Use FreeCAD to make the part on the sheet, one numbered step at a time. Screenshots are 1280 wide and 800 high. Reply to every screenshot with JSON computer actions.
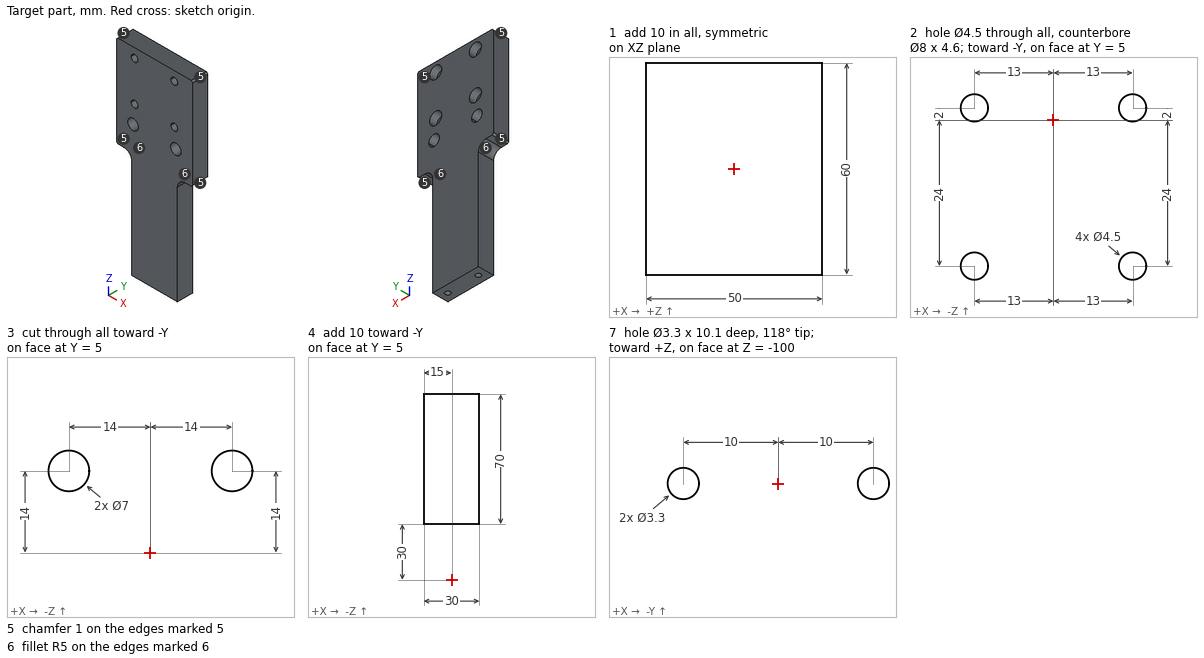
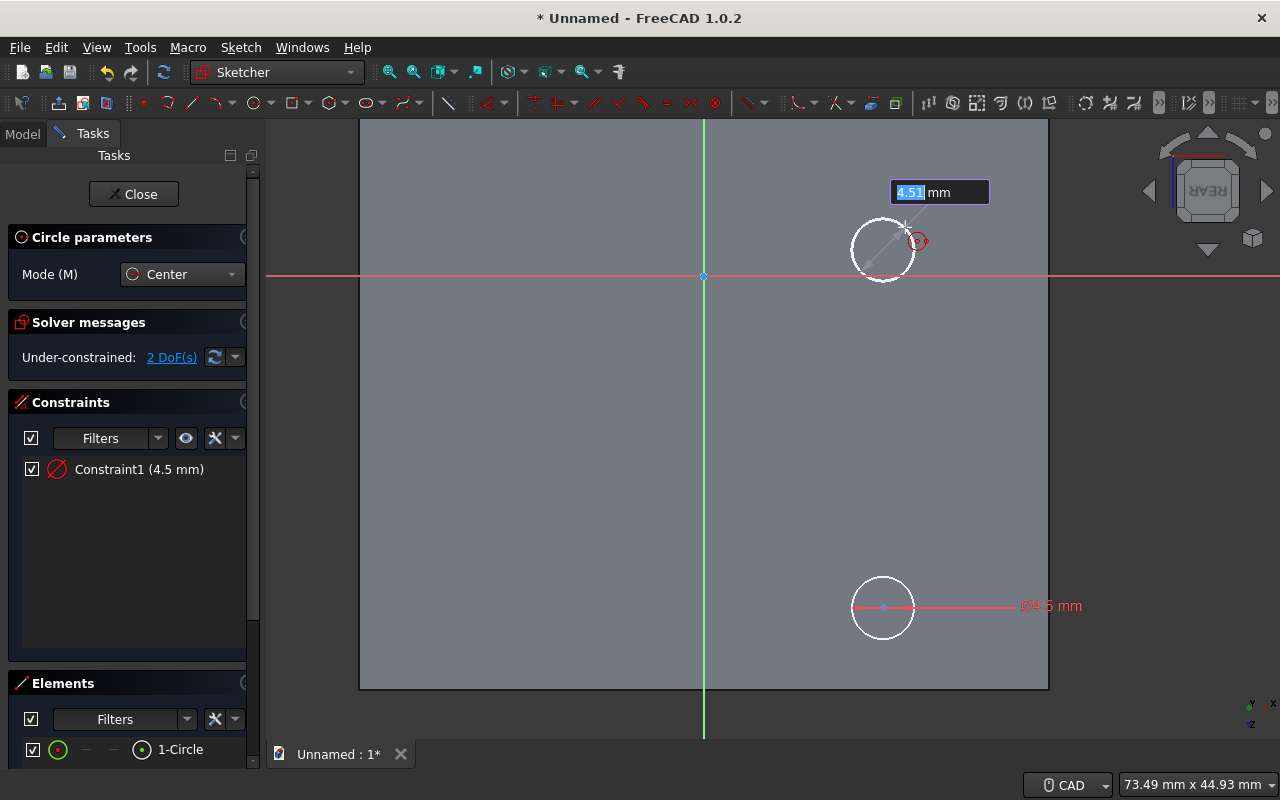
{"action": "type", "text": "4.5"}
{"action": "key", "text": "Return"}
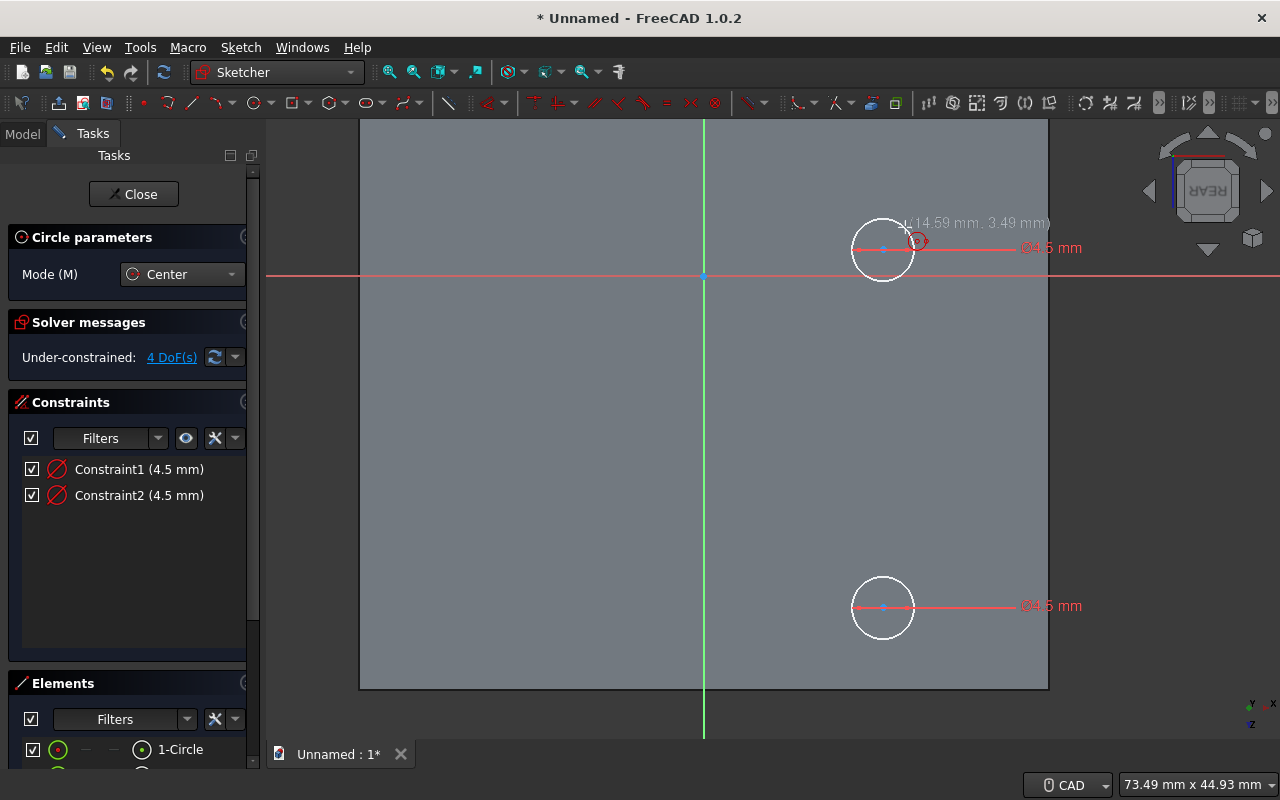
{"action": "left_click", "coordinate": [524, 249]}
{"action": "mouse_move", "coordinate": [546, 227]}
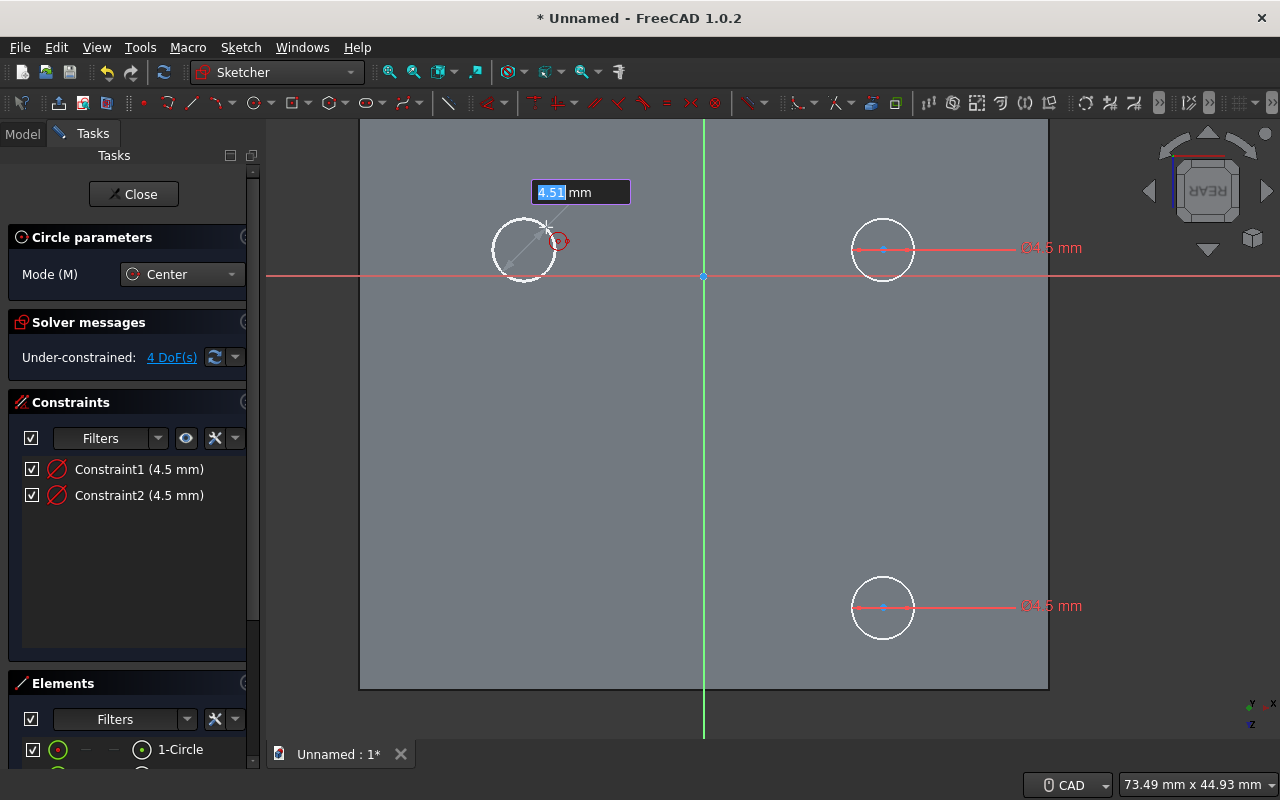
{"action": "type", "text": "4.5"}
{"action": "key", "text": "Return"}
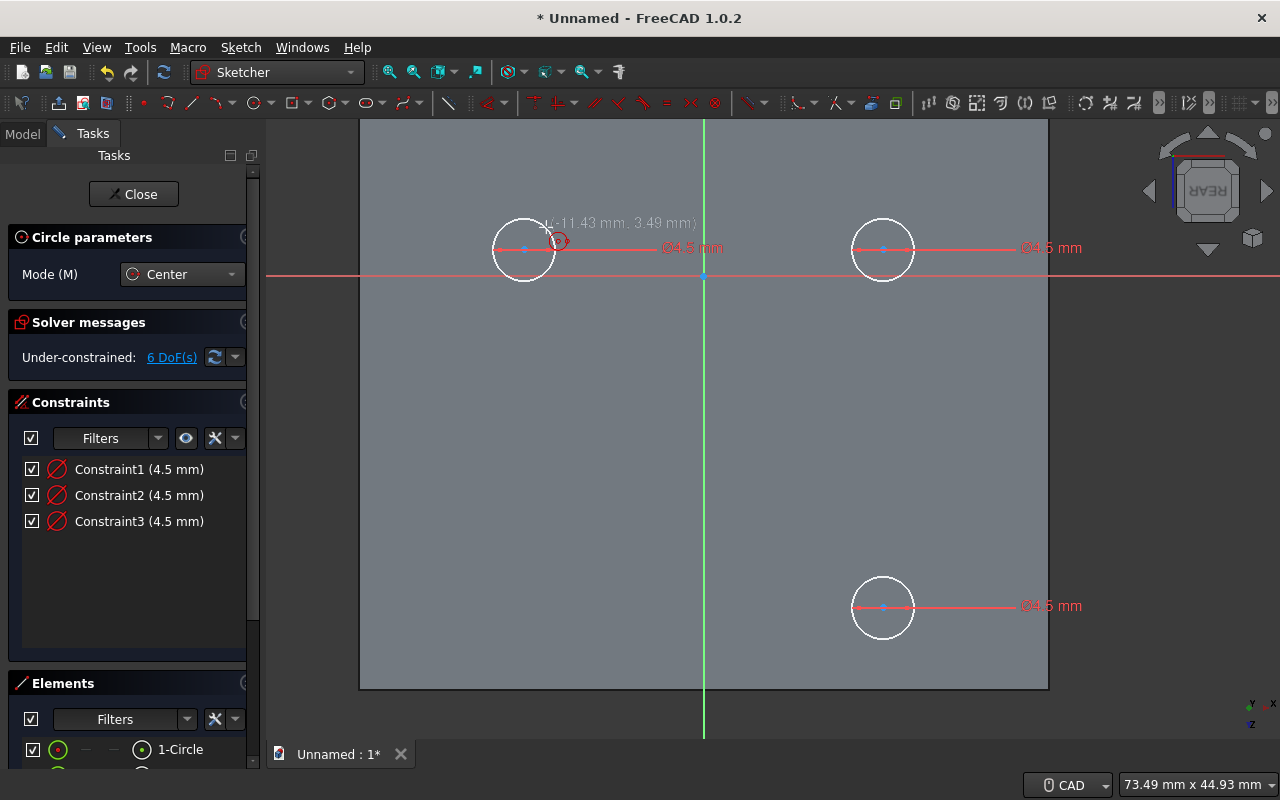
{"action": "left_click", "coordinate": [524, 607]}
{"action": "mouse_move", "coordinate": [546, 585]}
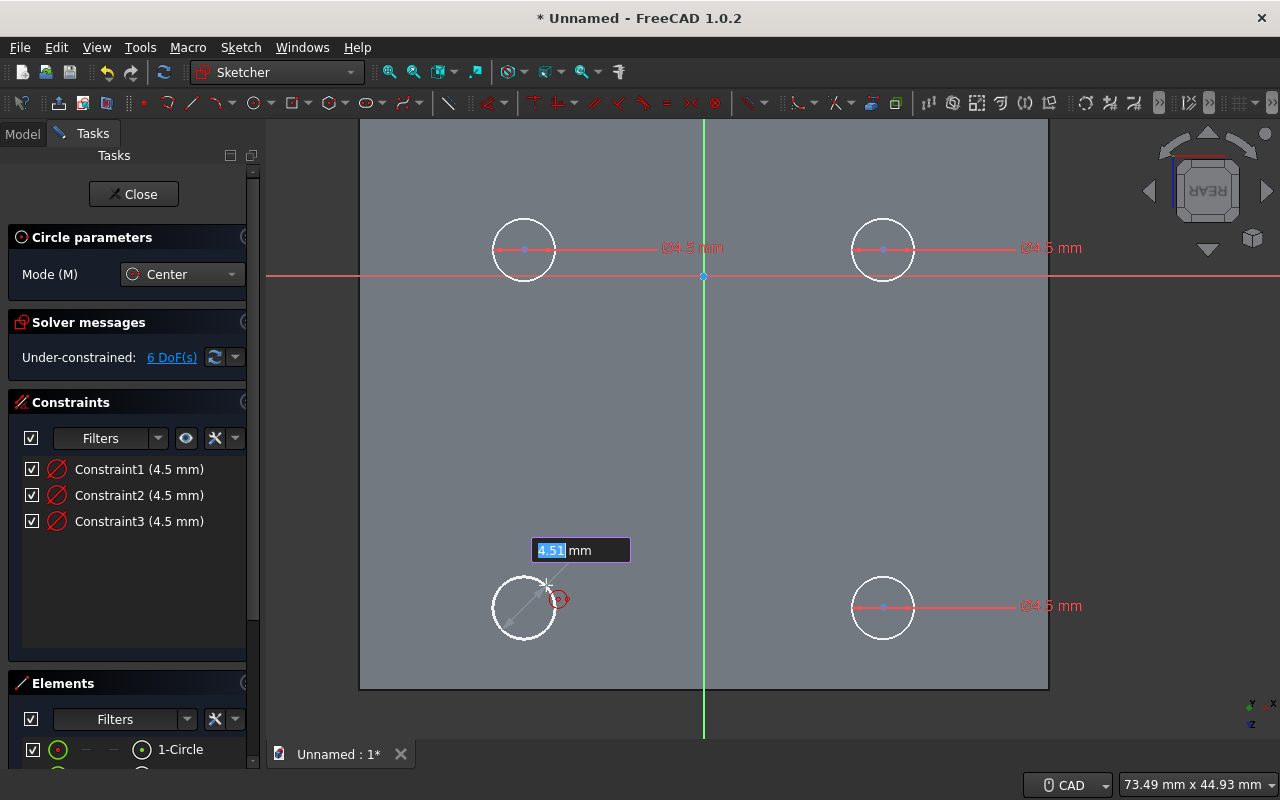
{"action": "type", "text": "4.5"}
{"action": "key", "text": "Return"}
{"action": "key", "text": "Escape"}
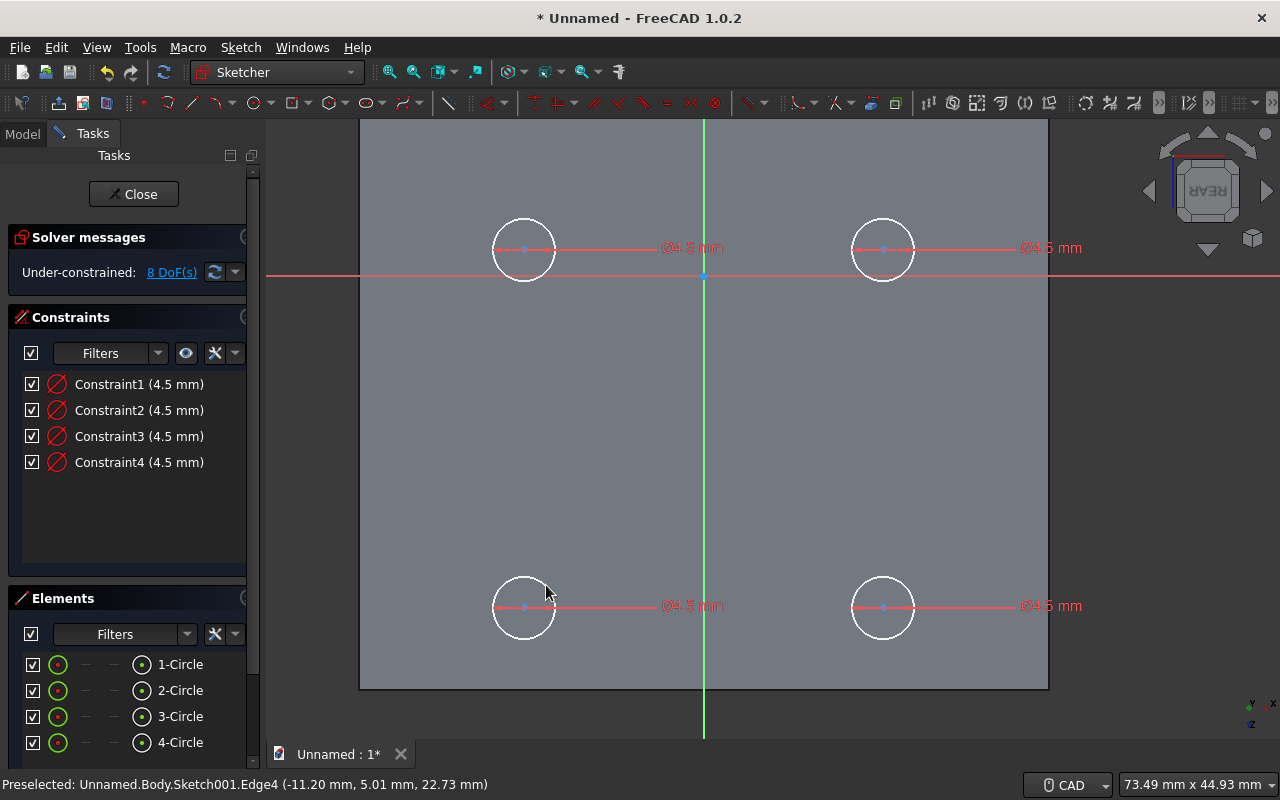
{"action": "key", "text": "d"}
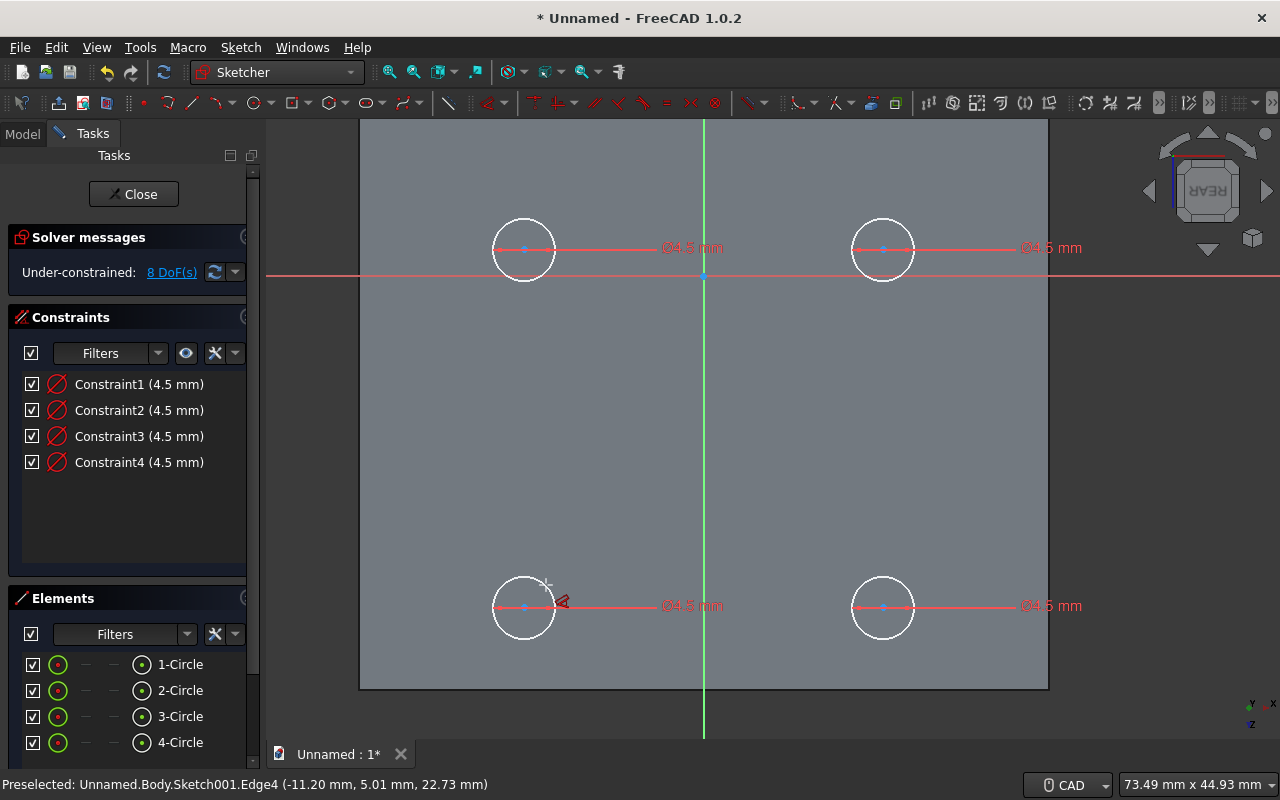
{"action": "scroll", "coordinate": [883, 250], "scroll_direction": "up", "scroll_amount": 2}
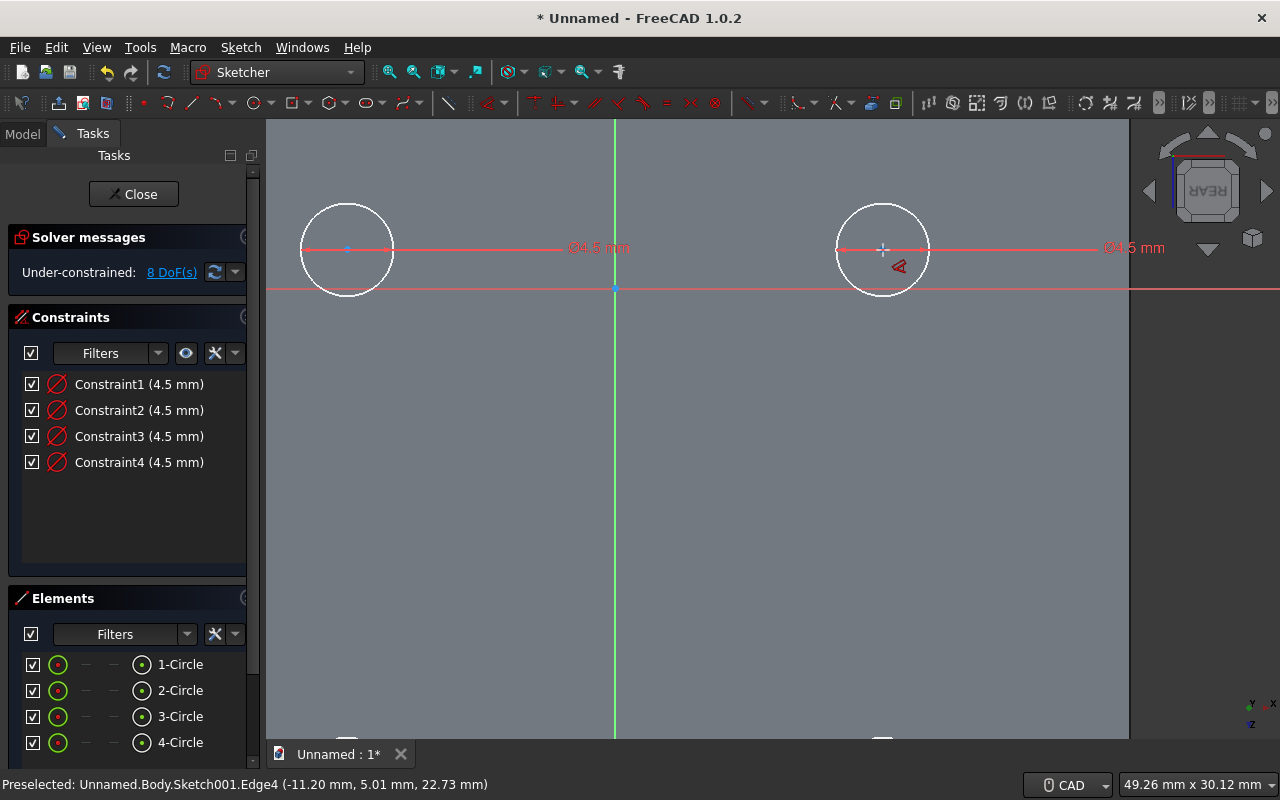
{"action": "left_click", "coordinate": [883, 250]}
{"action": "left_click", "coordinate": [581, 269]}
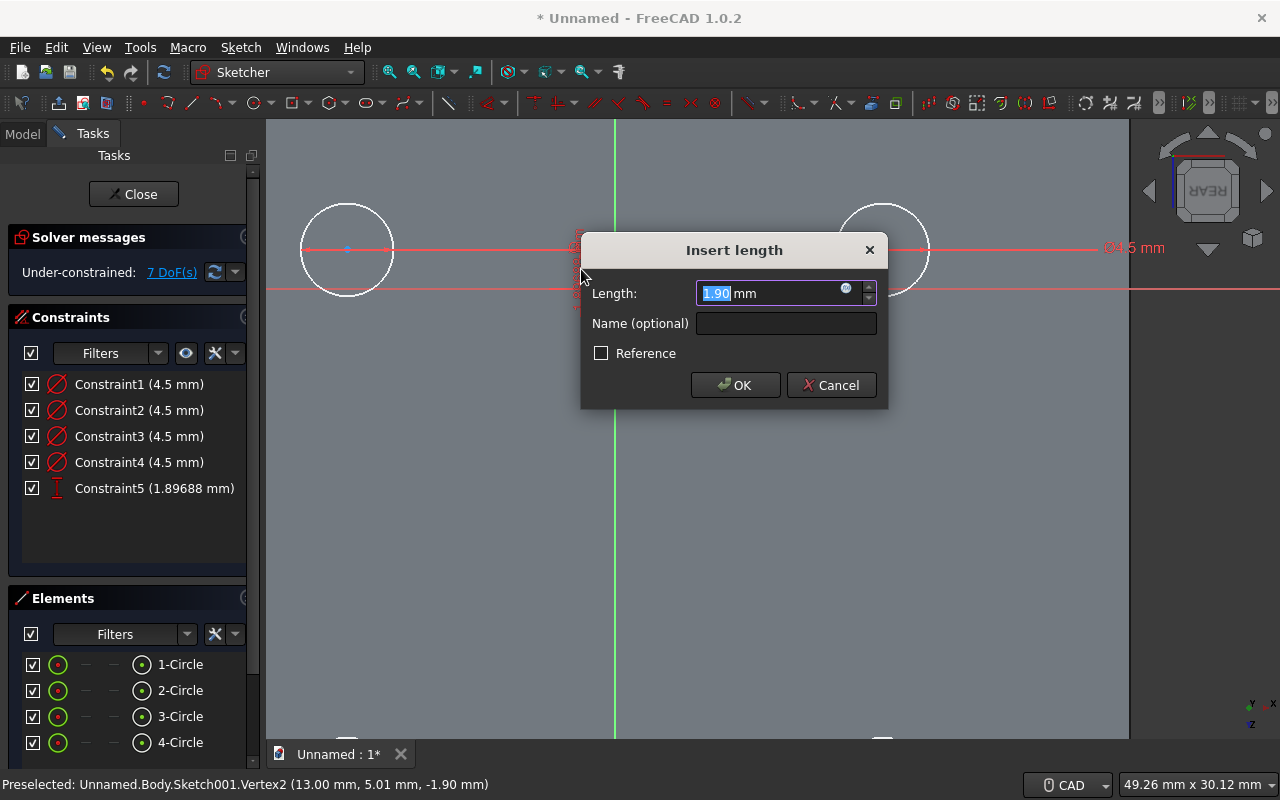
{"action": "type", "text": "2"}
{"action": "key", "text": "Return"}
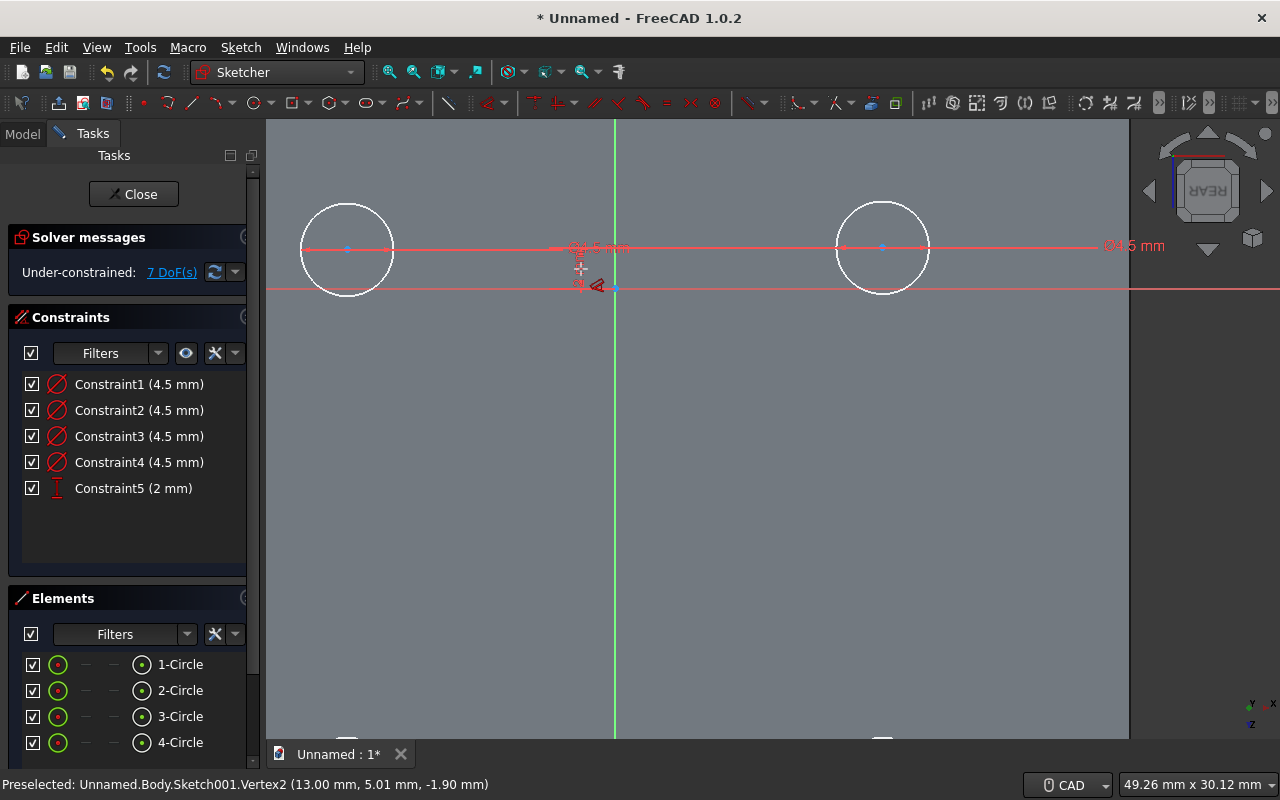
{"action": "left_click", "coordinate": [347, 250]}
{"action": "left_click", "coordinate": [673, 269]}